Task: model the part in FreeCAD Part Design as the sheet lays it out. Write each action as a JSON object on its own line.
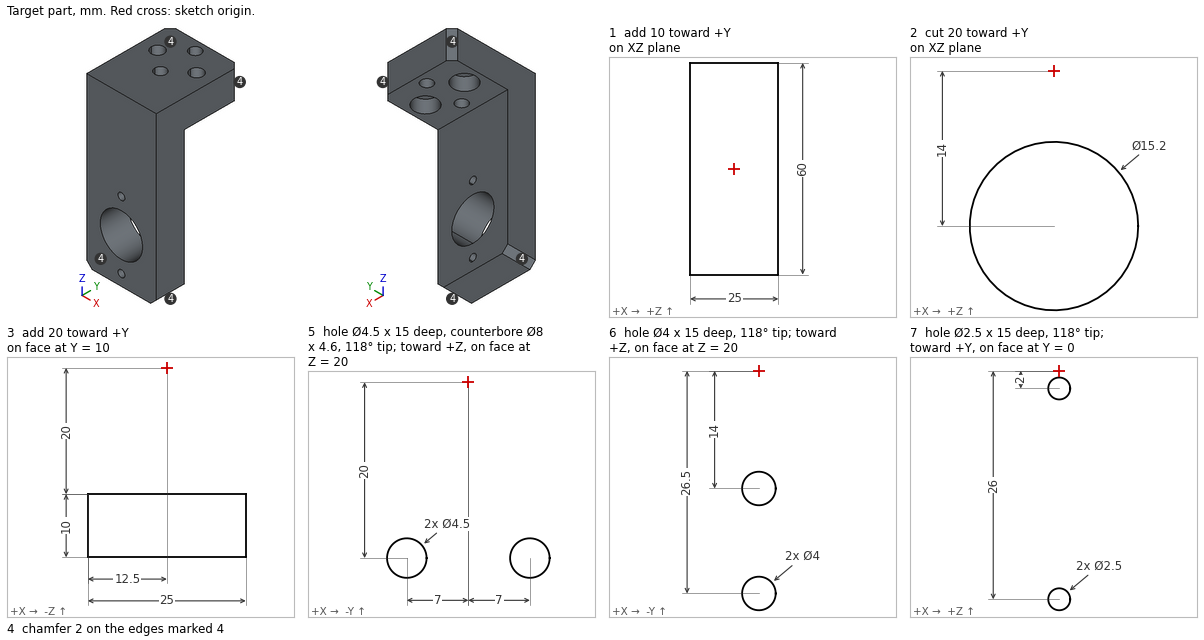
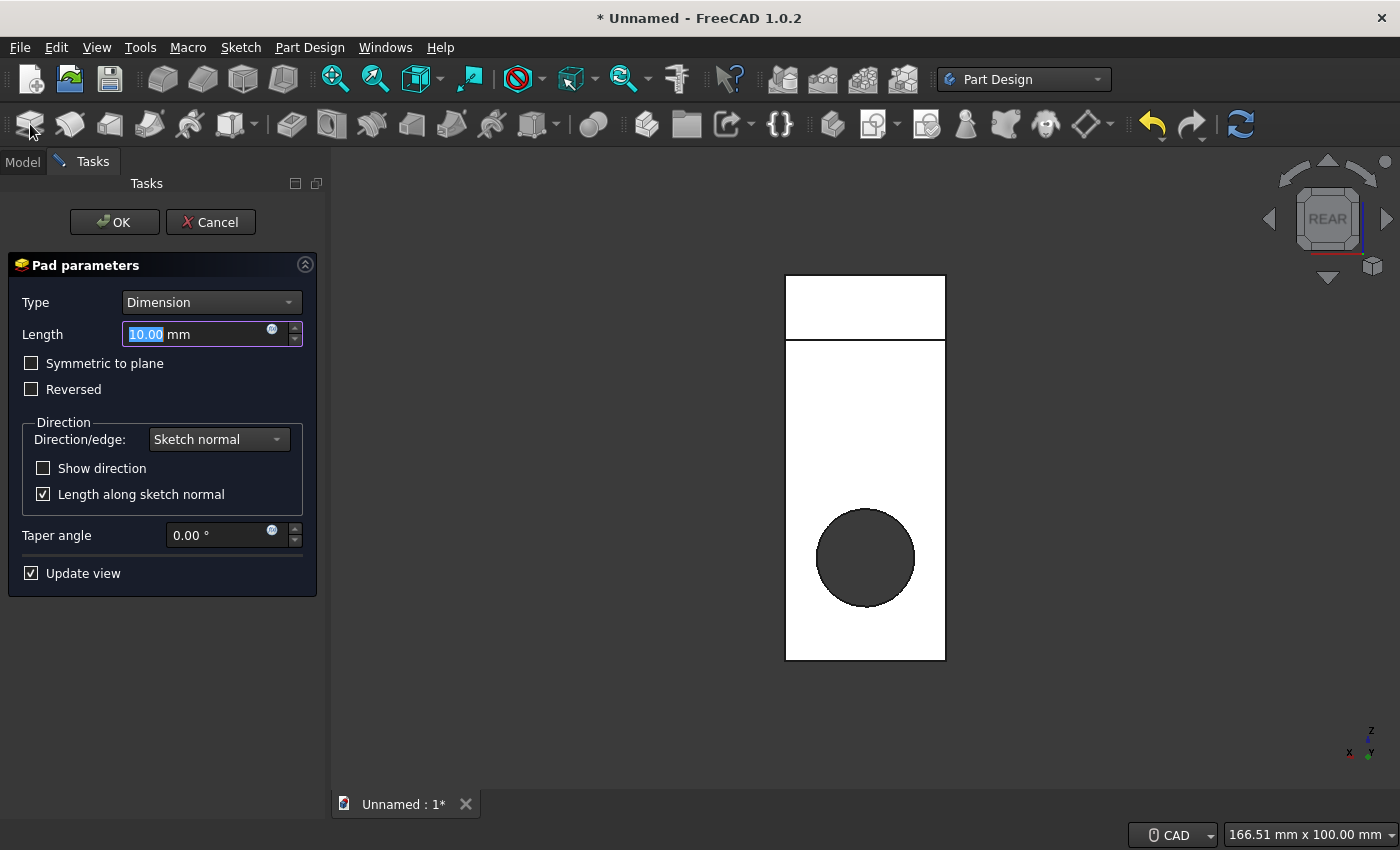
{"action": "type", "text": "20"}
{"action": "key", "text": "Tab"}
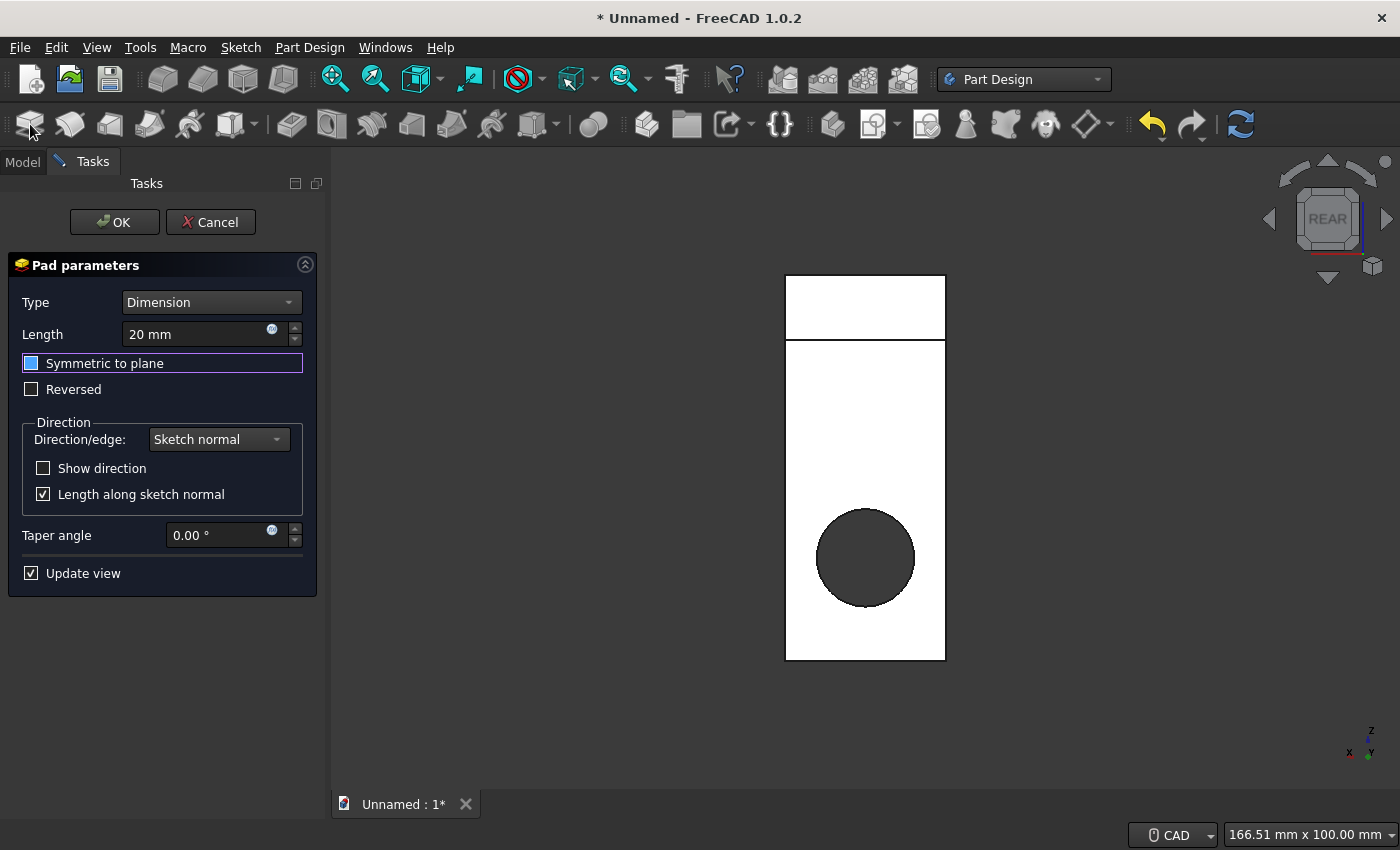
{"action": "left_click", "coordinate": [115, 222]}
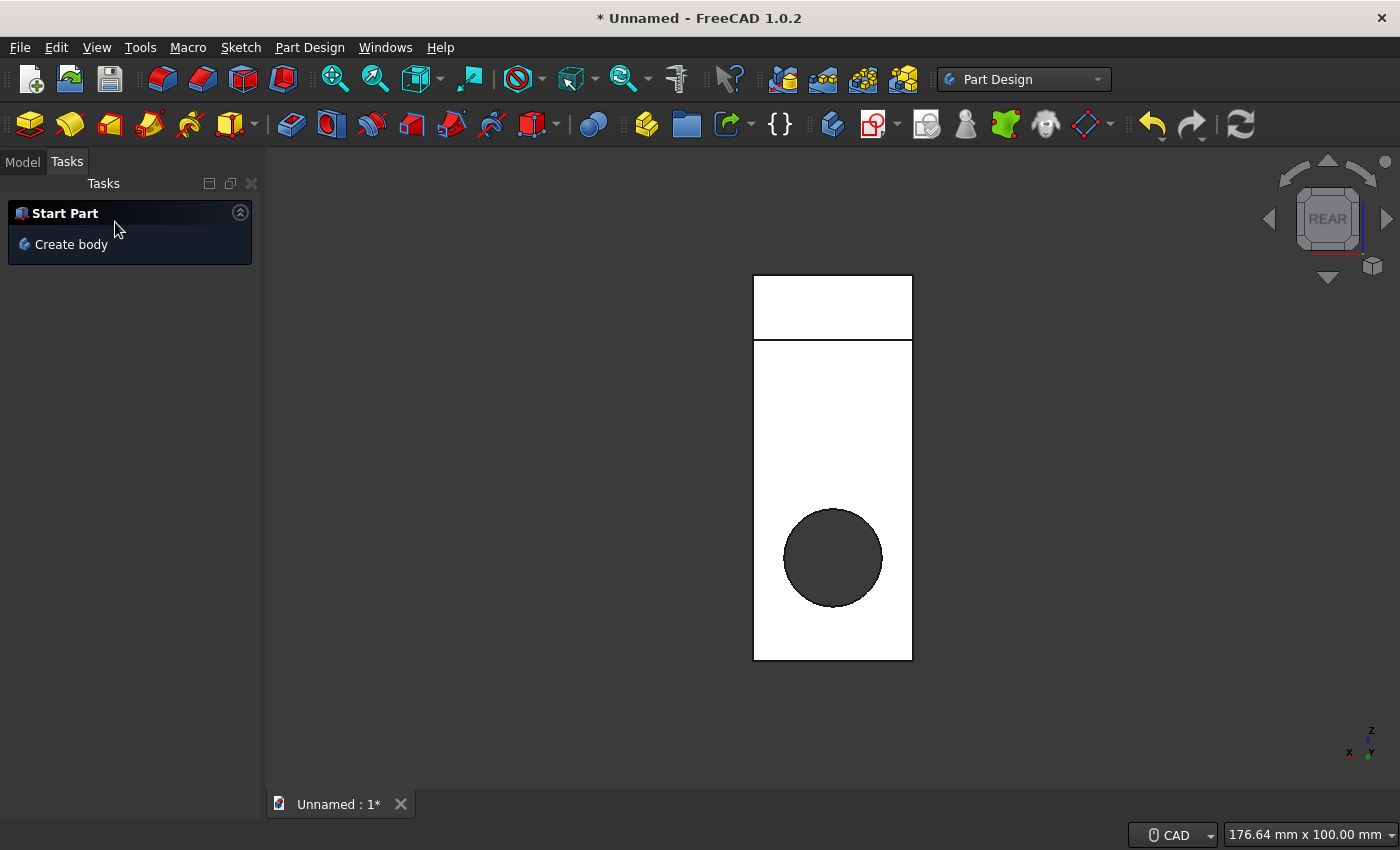
{"action": "left_click", "coordinate": [913, 306]}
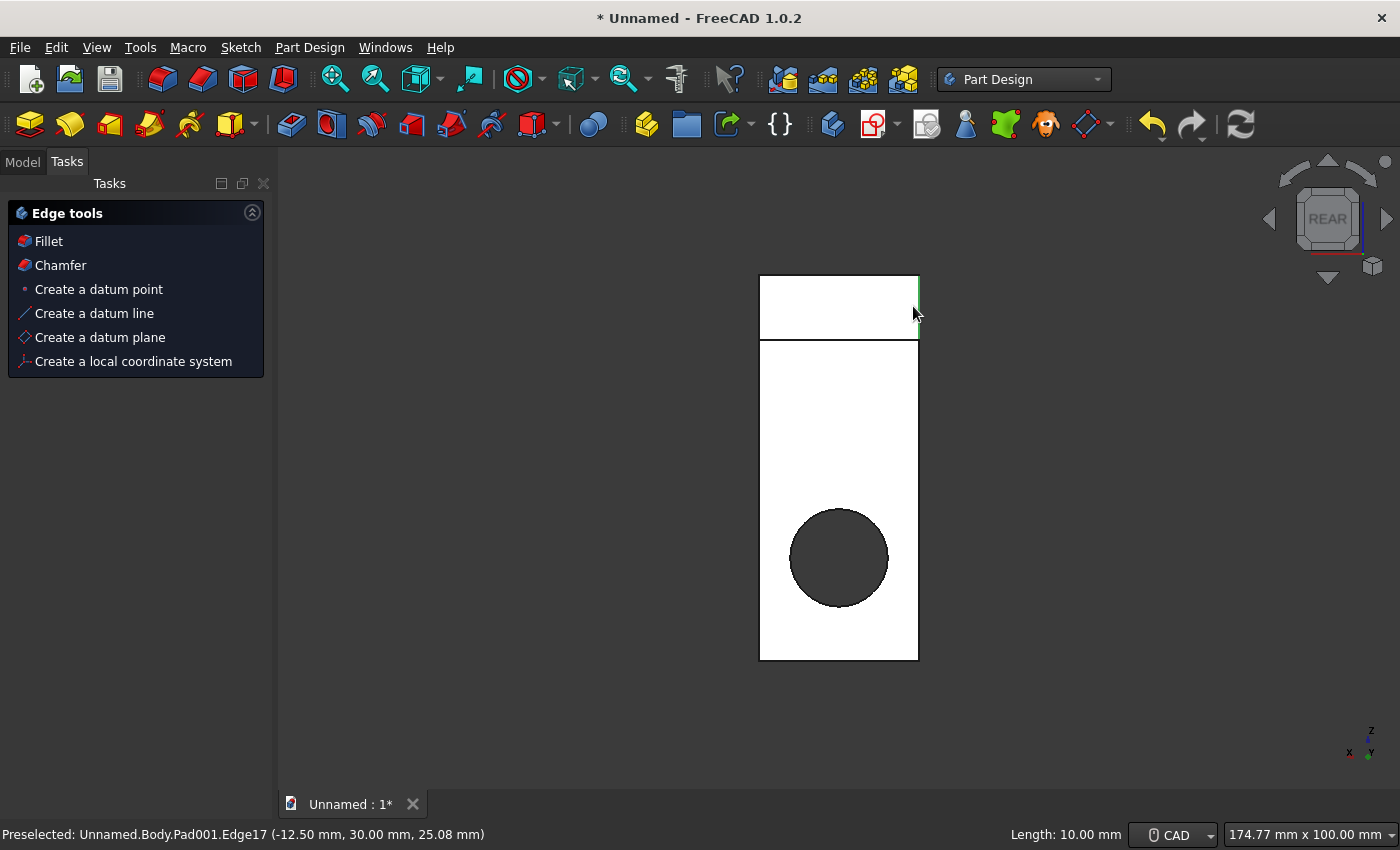
{"action": "key", "text": "0"}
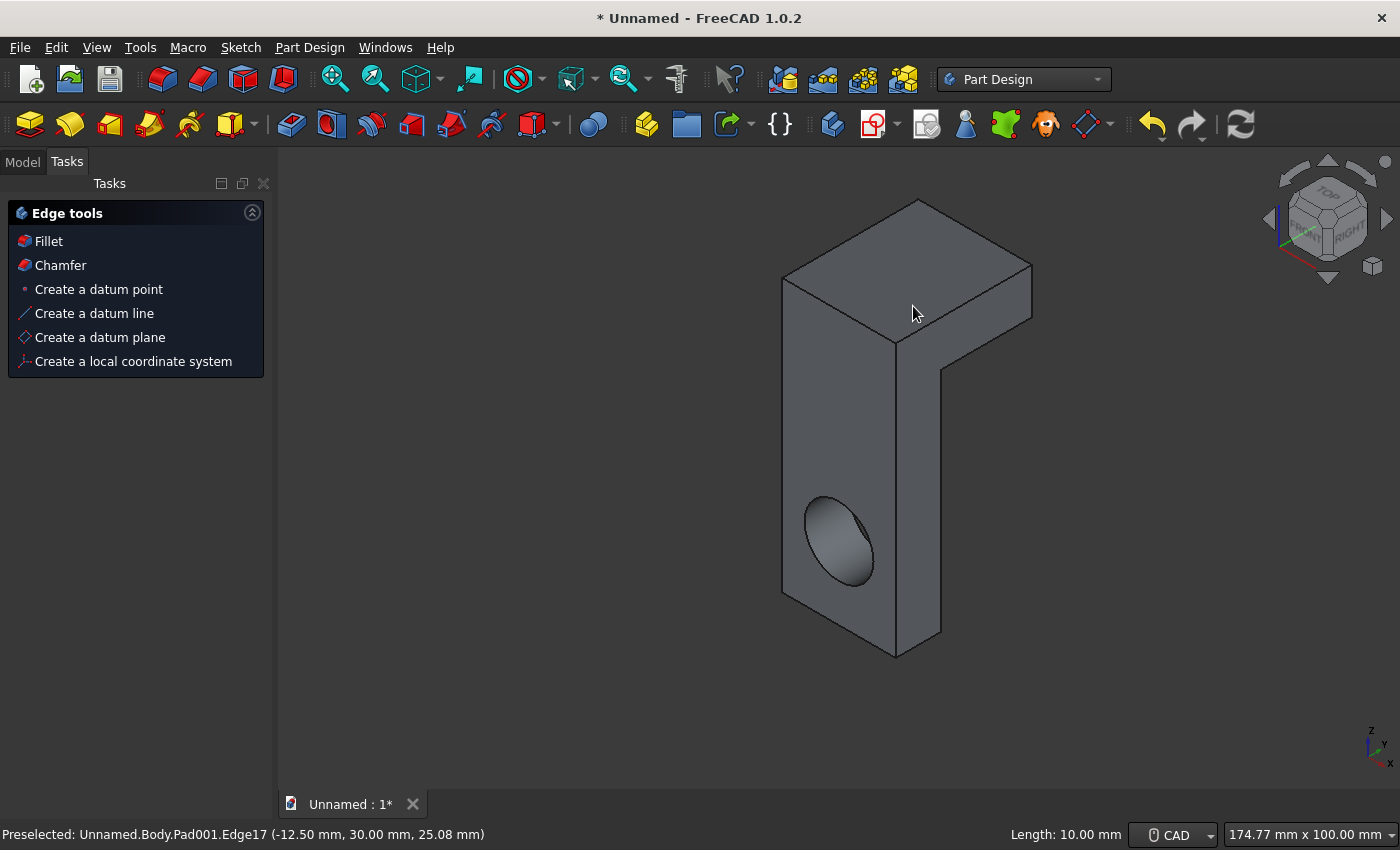
{"action": "key", "text": "2"}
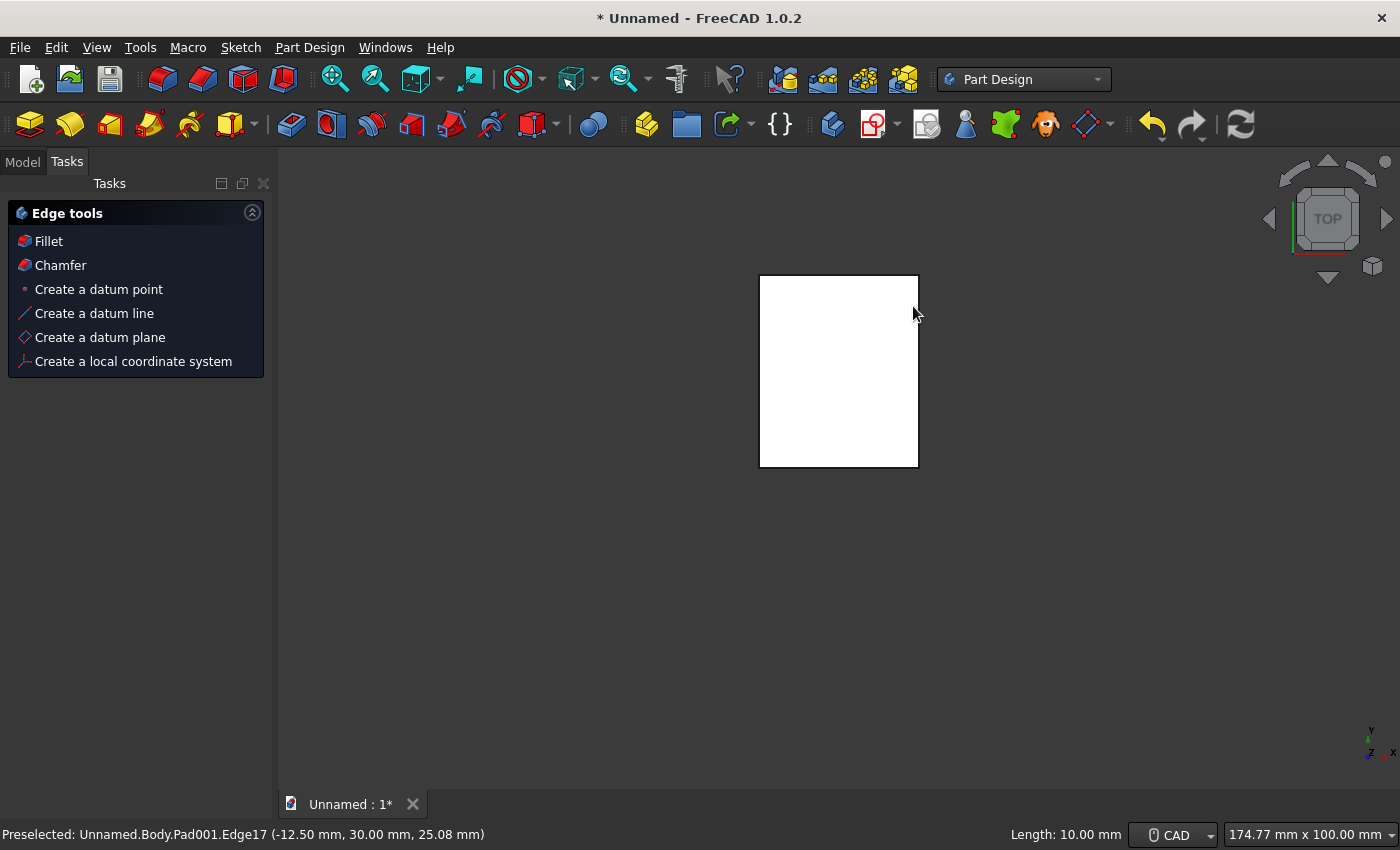
{"action": "key", "text": "v f"}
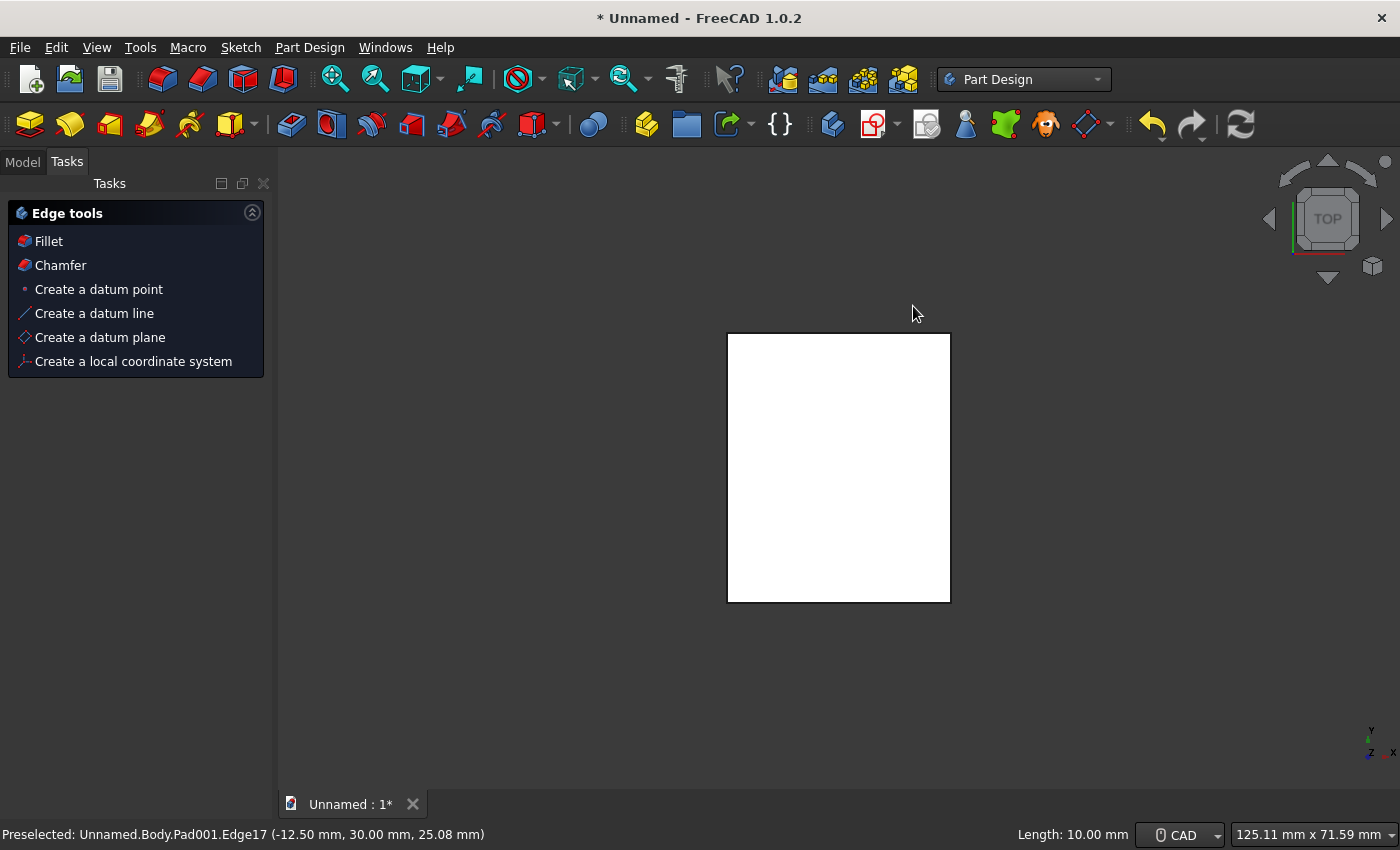
{"action": "key", "text": "1"}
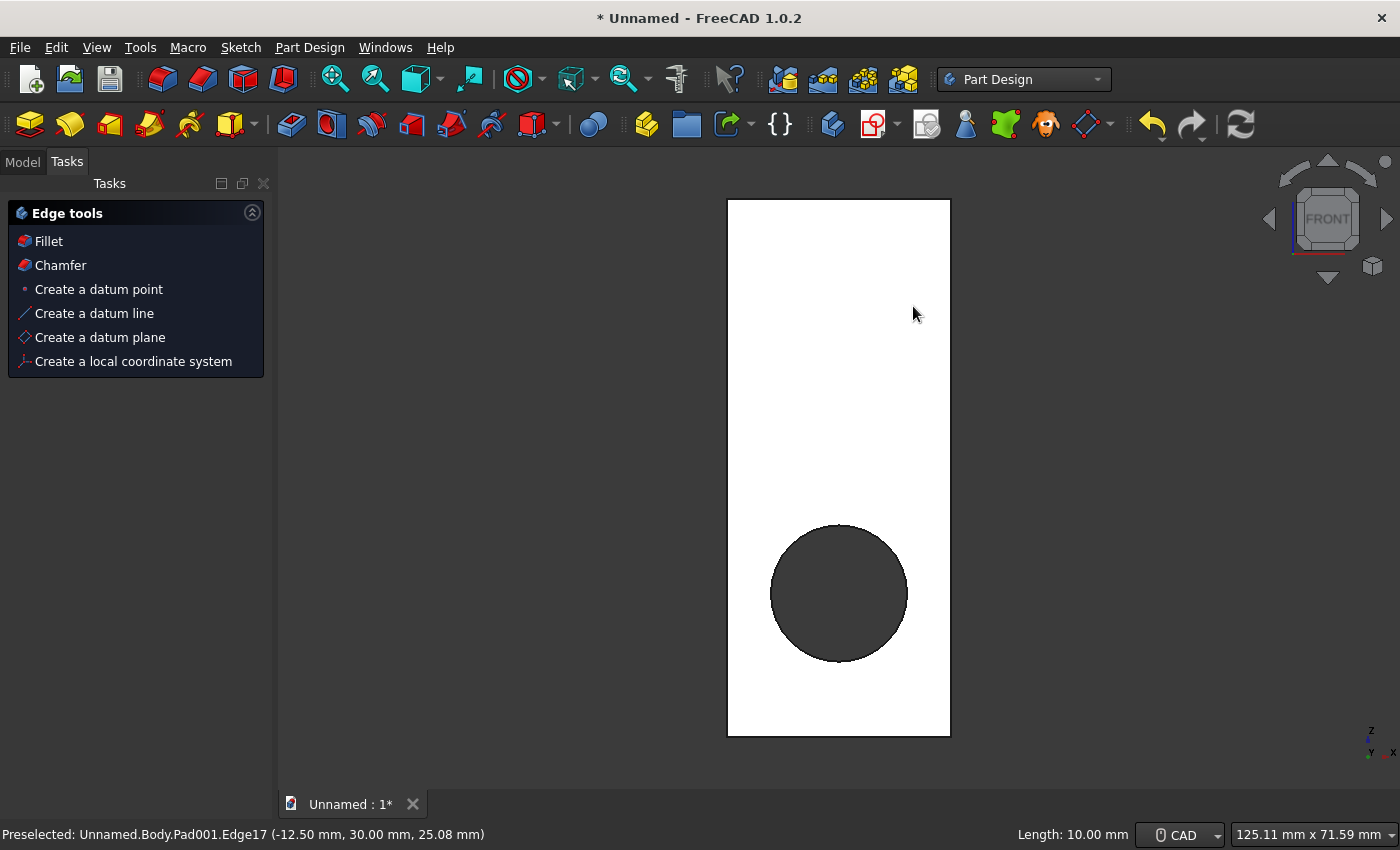
{"action": "key", "text": "3"}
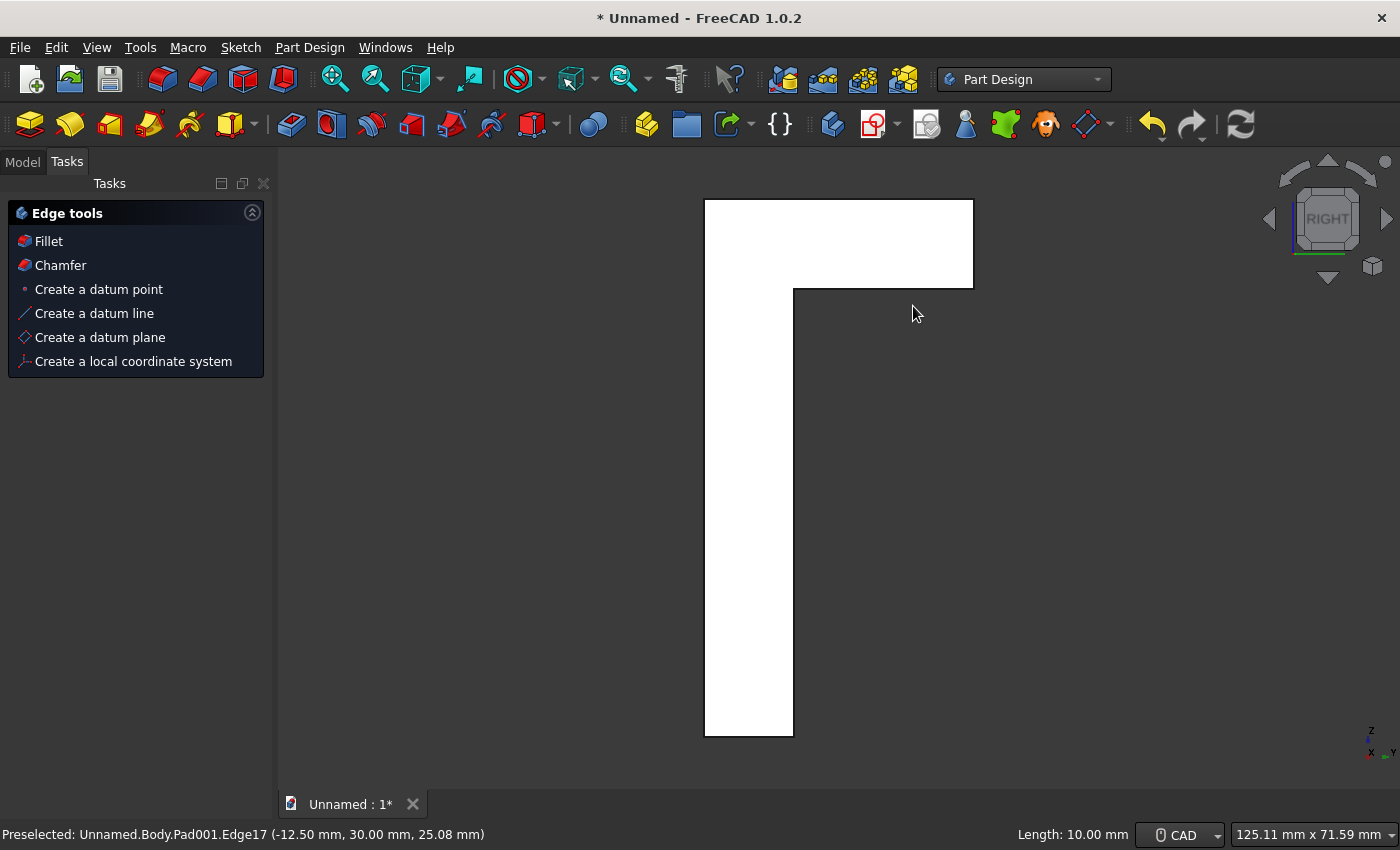
{"action": "left_click", "coordinate": [974, 243], "text": "ctrl"}